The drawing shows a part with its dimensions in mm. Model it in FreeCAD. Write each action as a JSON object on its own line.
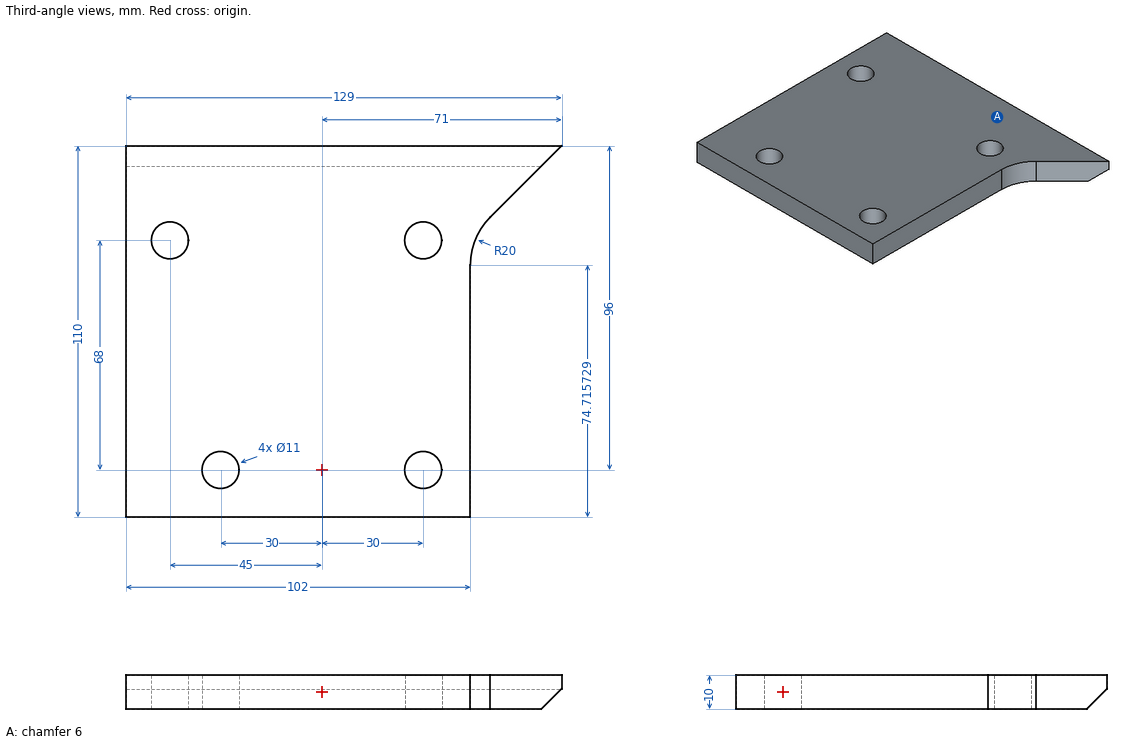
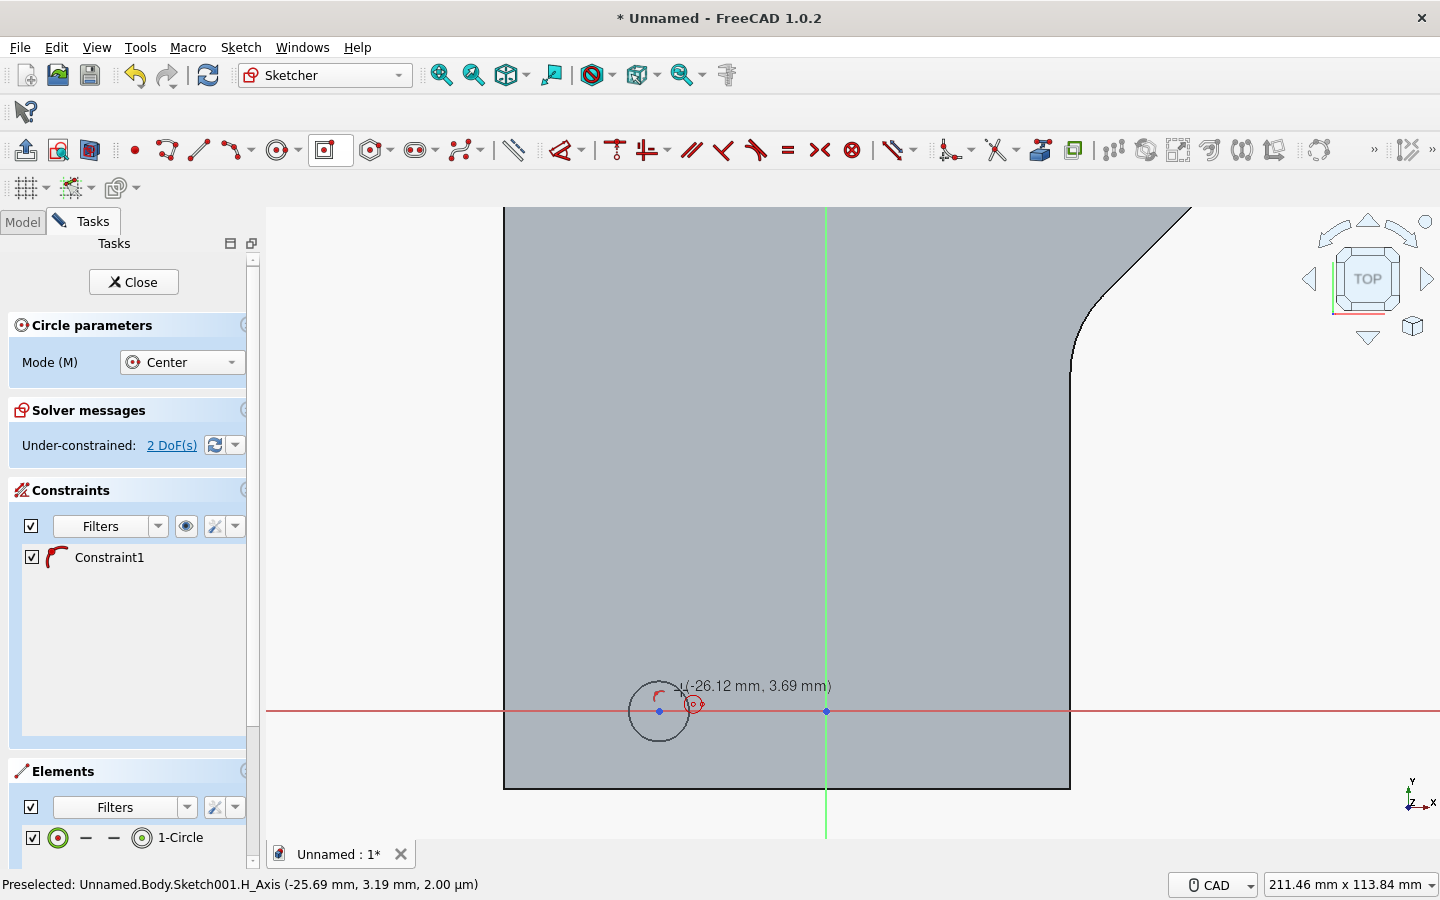
{"action": "left_click", "coordinate": [993, 711]}
{"action": "left_click", "coordinate": [1014, 690]}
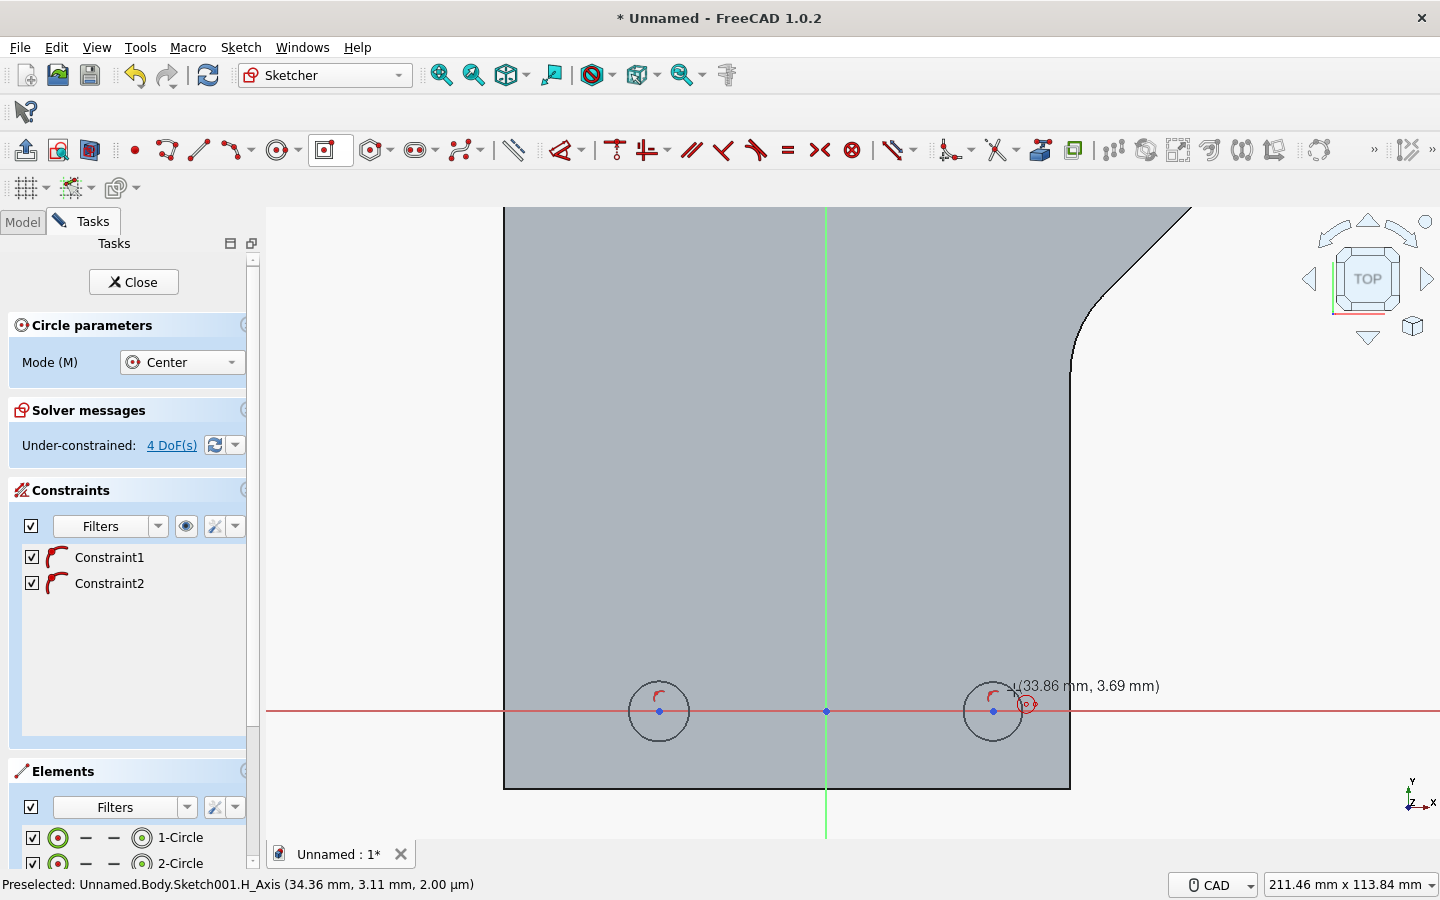
{"action": "left_click", "coordinate": [576, 334]}
{"action": "left_click", "coordinate": [598, 312]}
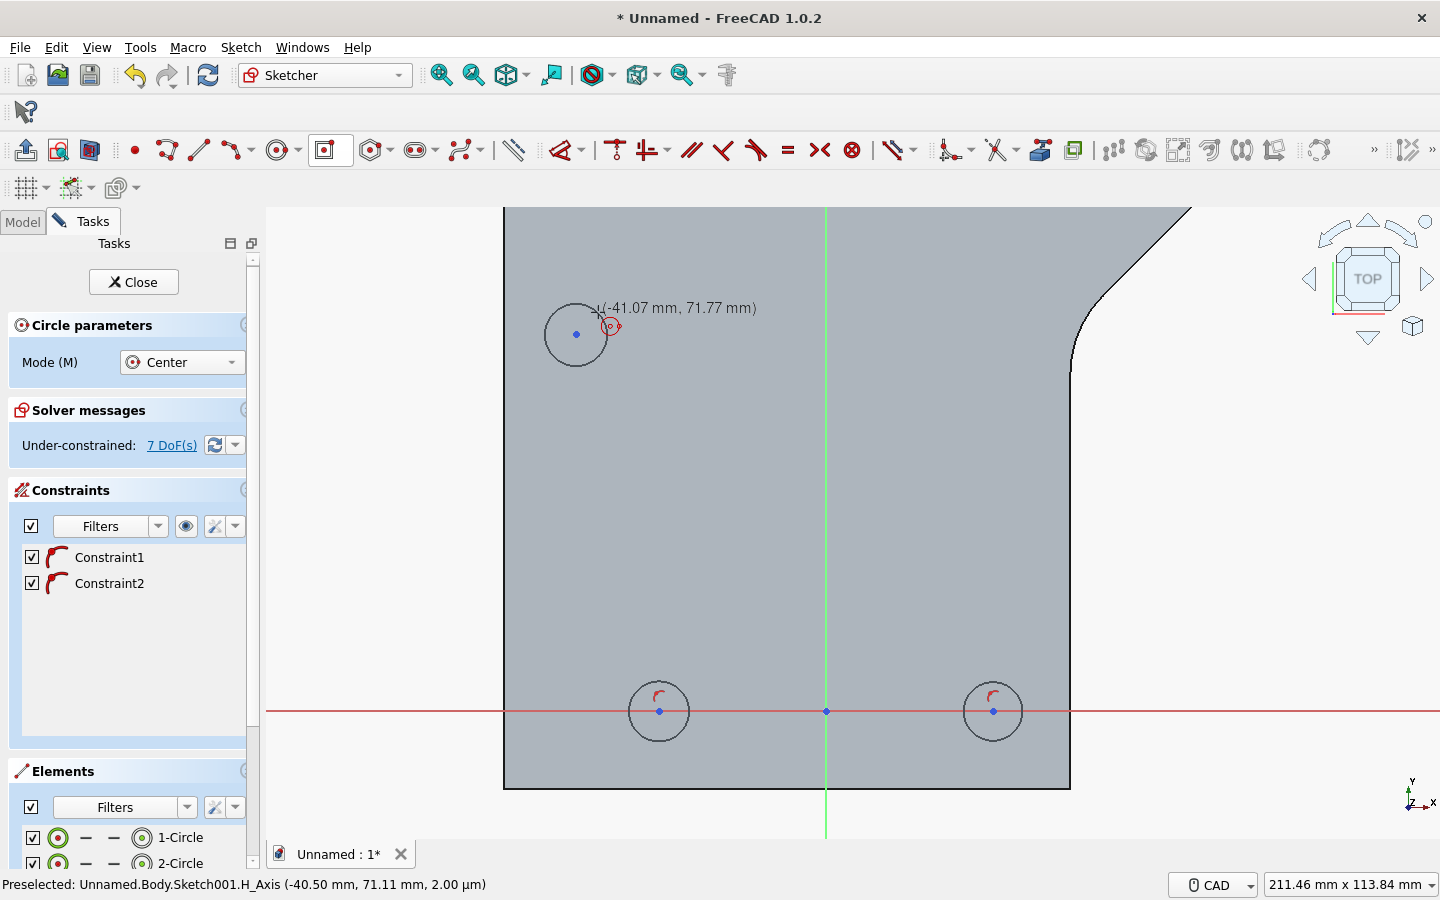
{"action": "left_click", "coordinate": [993, 334]}
{"action": "left_click", "coordinate": [1014, 312]}
{"action": "key", "text": "Escape"}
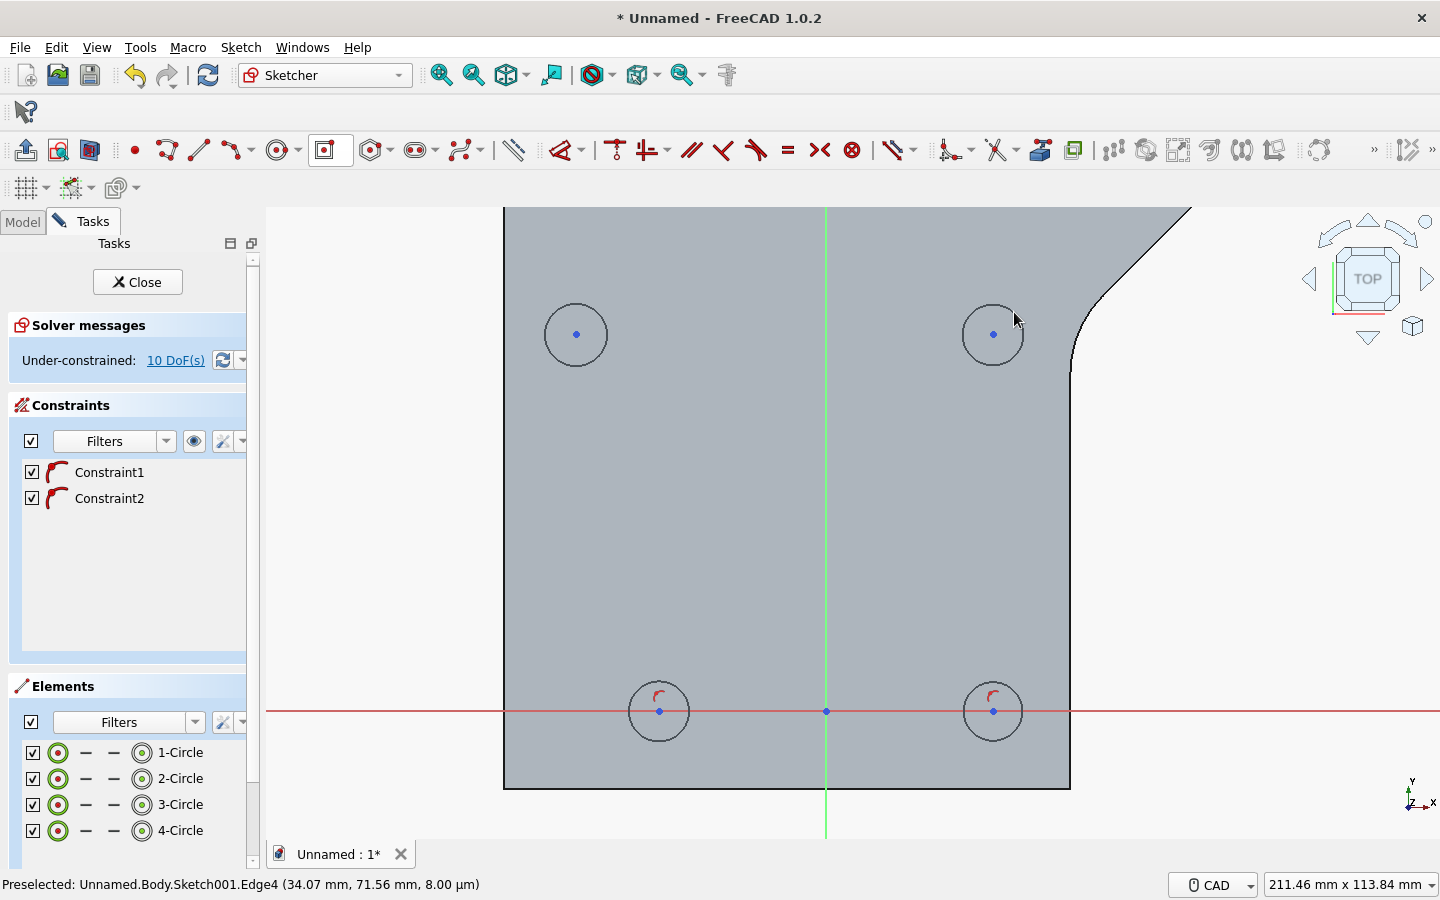
{"action": "left_click", "coordinate": [680, 690]}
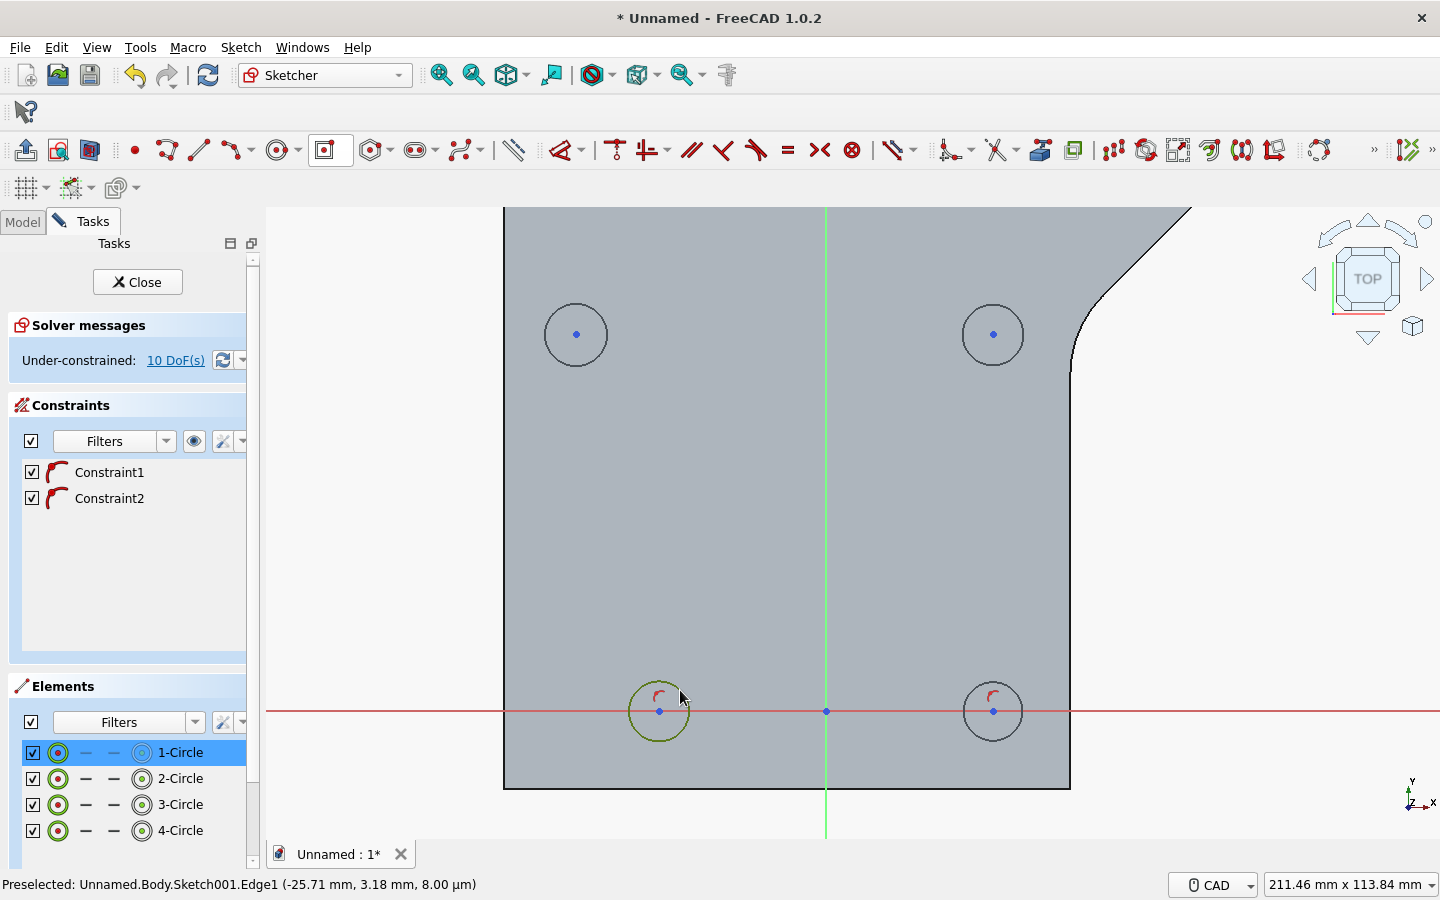
{"action": "left_click", "coordinate": [1014, 691]}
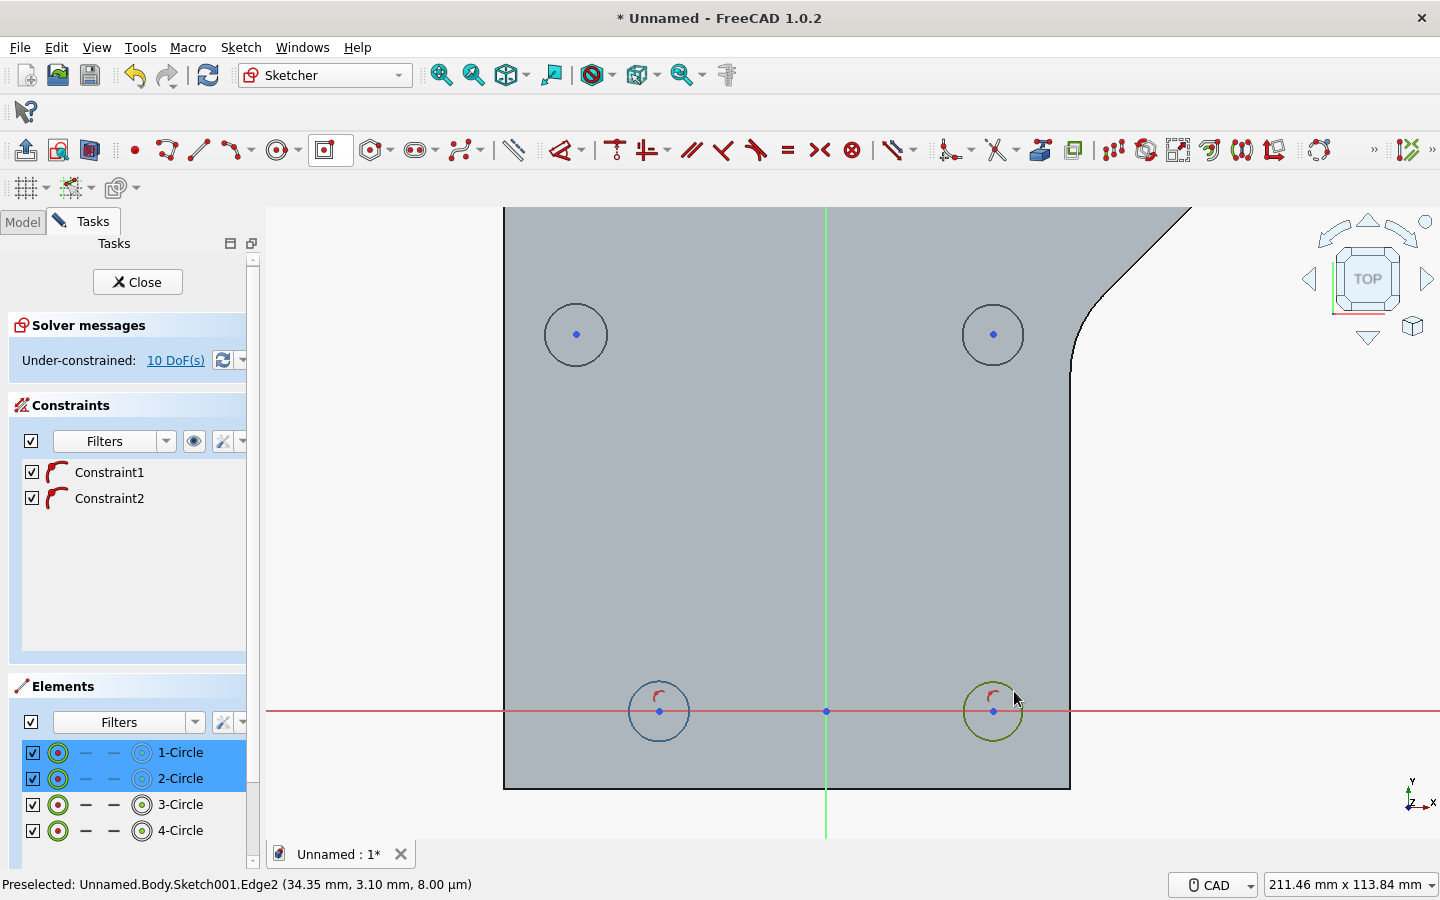
{"action": "left_click", "coordinate": [598, 313]}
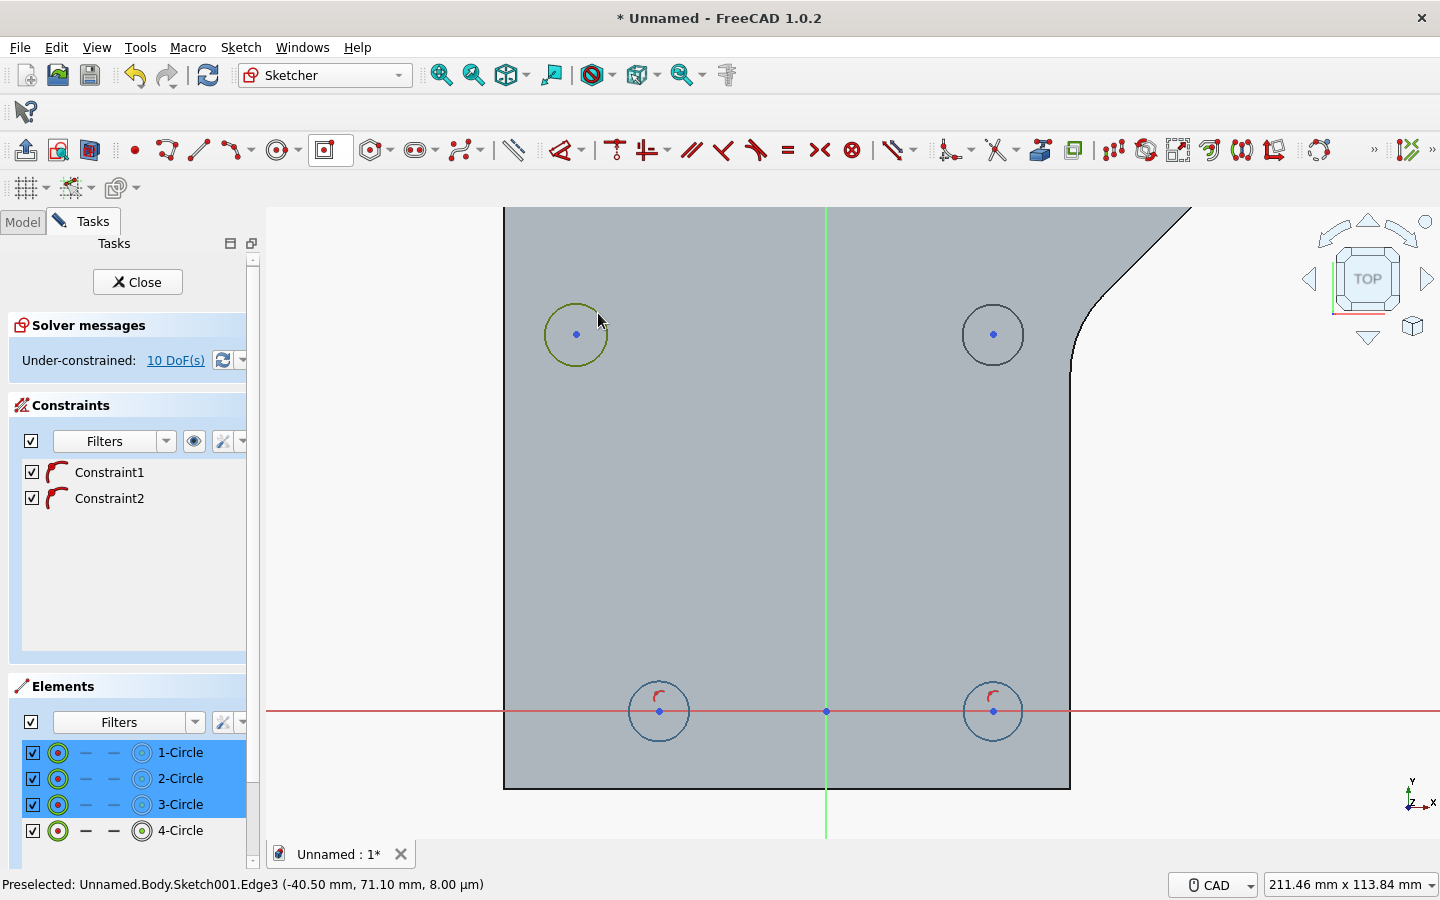
{"action": "left_click", "coordinate": [1014, 313]}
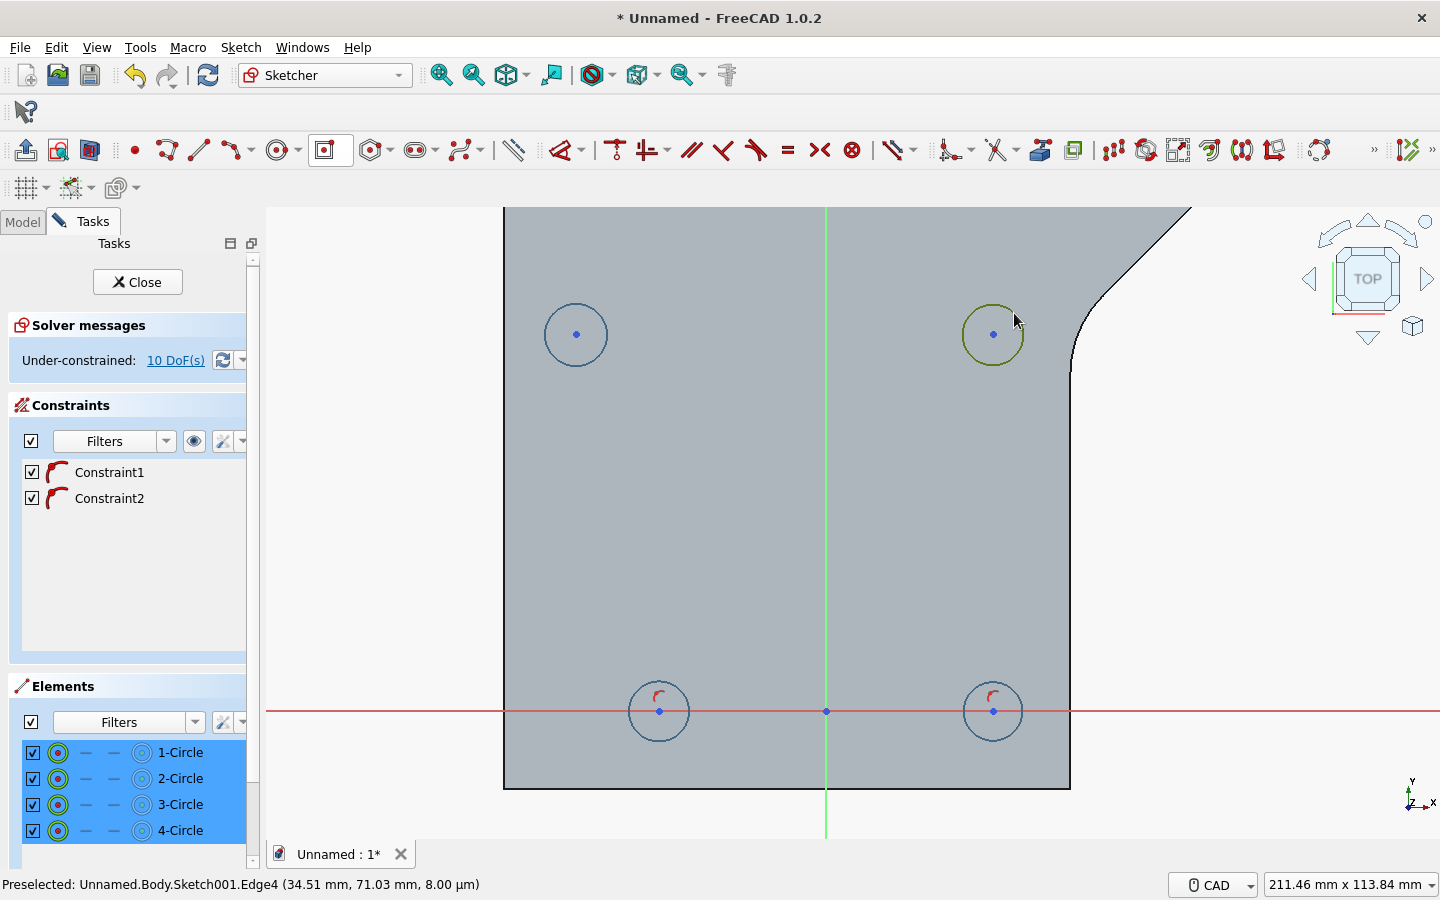
{"action": "left_click", "coordinate": [788, 150]}